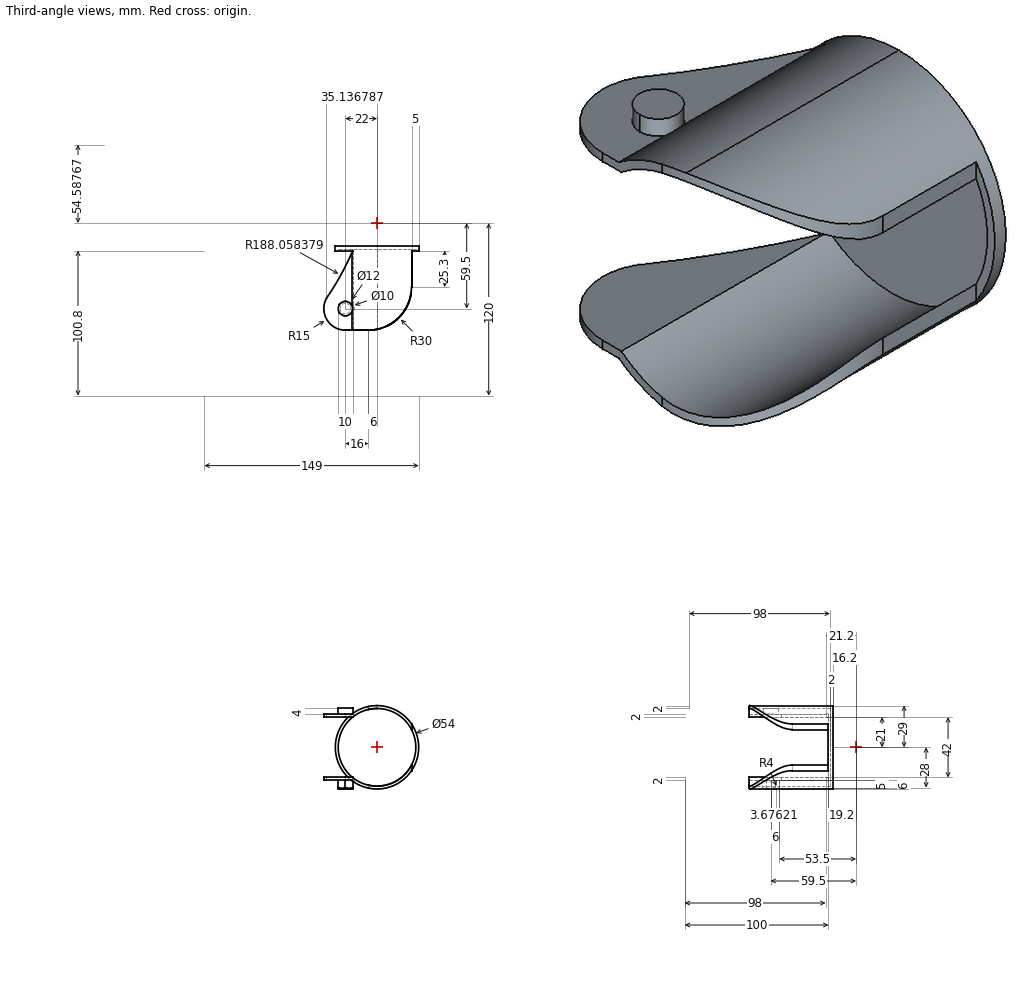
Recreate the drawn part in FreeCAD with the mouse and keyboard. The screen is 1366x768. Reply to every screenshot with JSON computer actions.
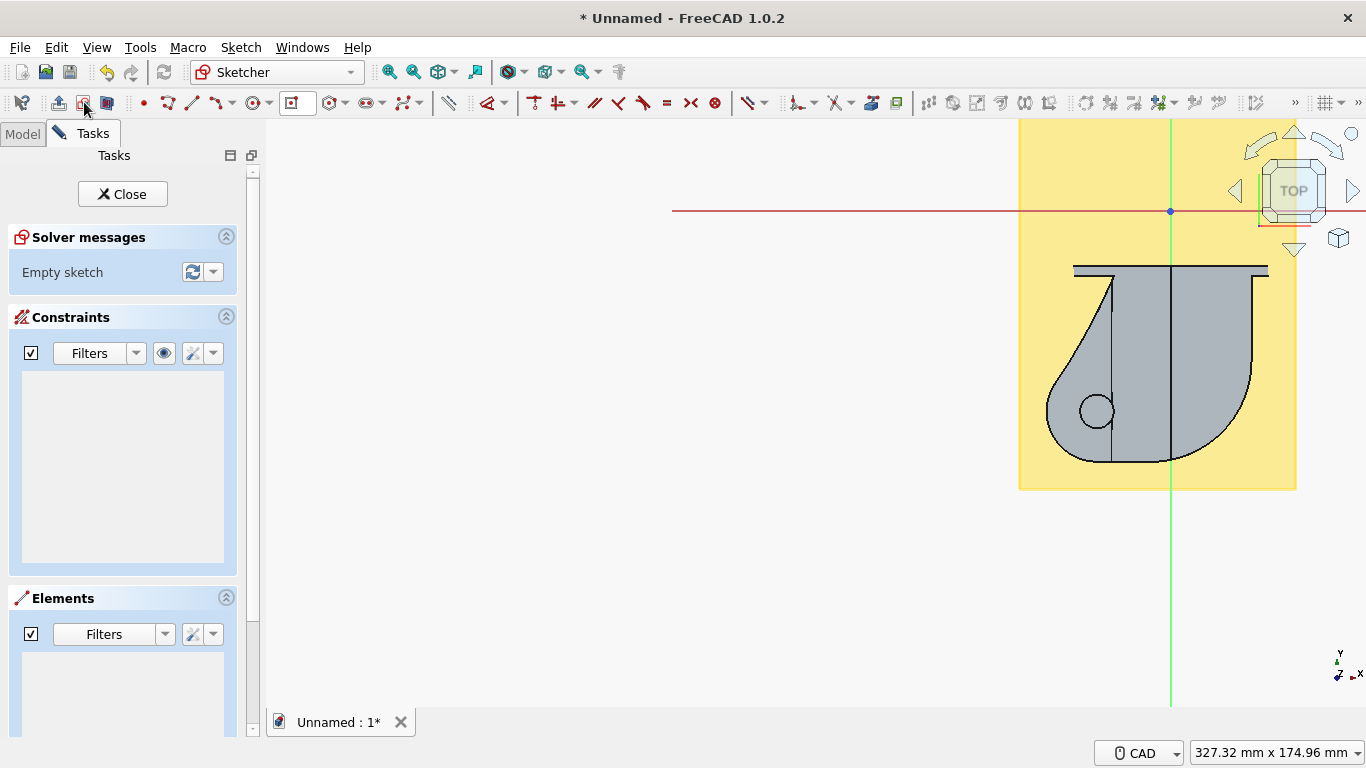
{"action": "left_click", "coordinate": [108, 104]}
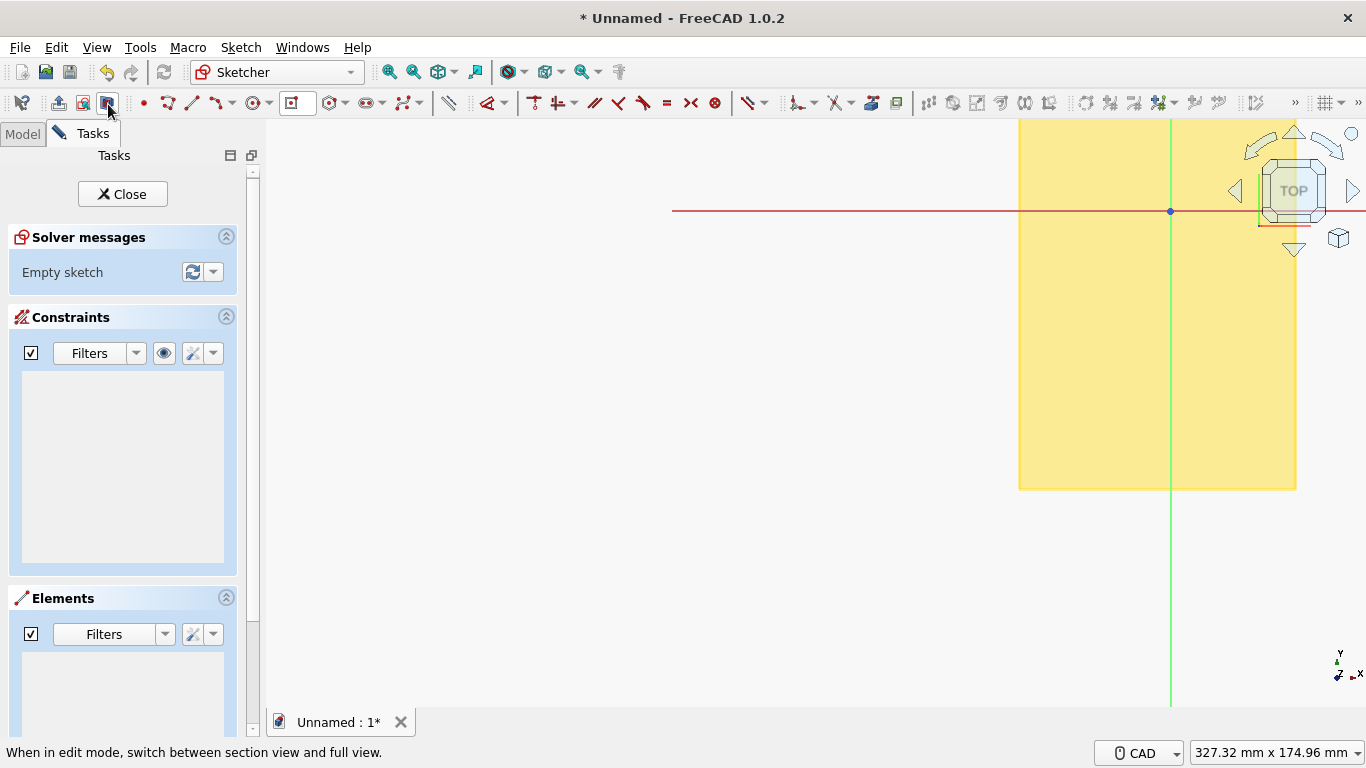
{"action": "scroll", "coordinate": [1140, 411], "scroll_direction": "up", "scroll_amount": 11}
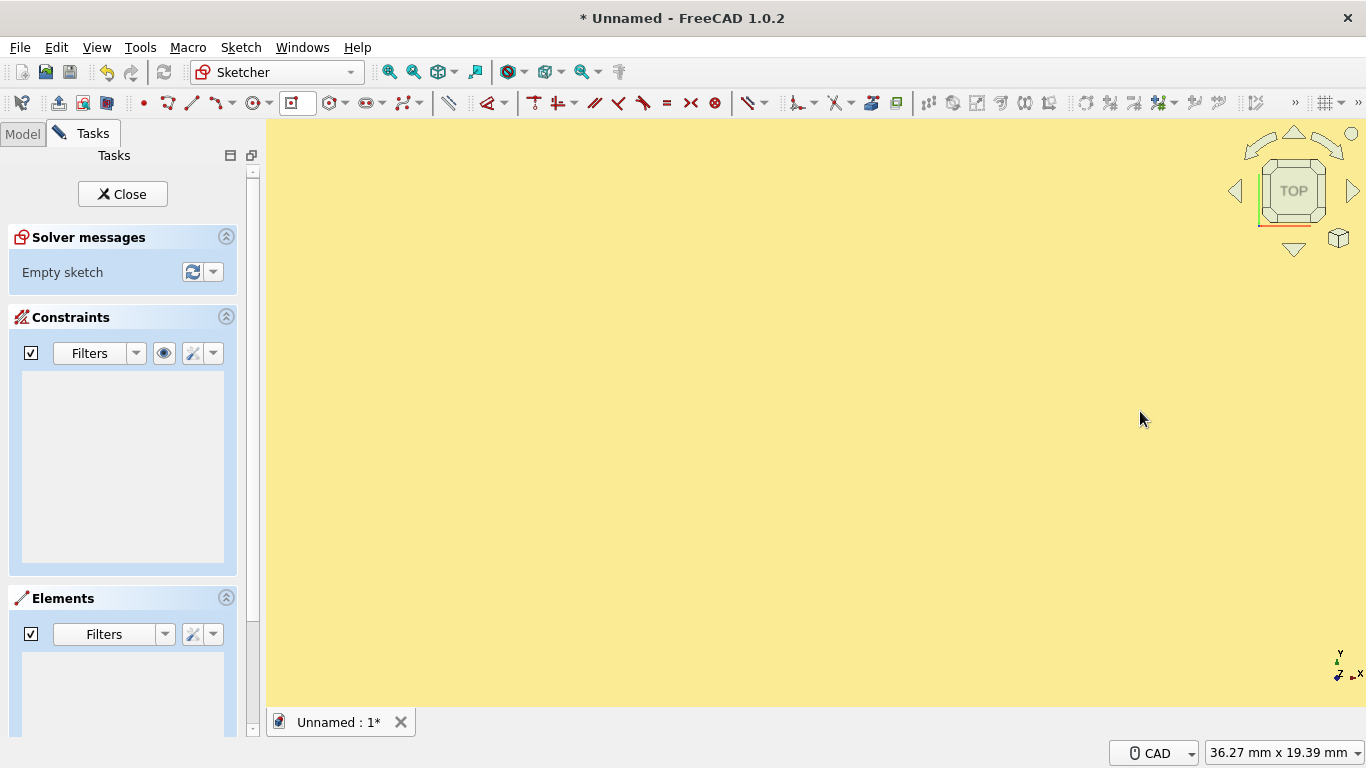
{"action": "left_click", "coordinate": [330, 104]}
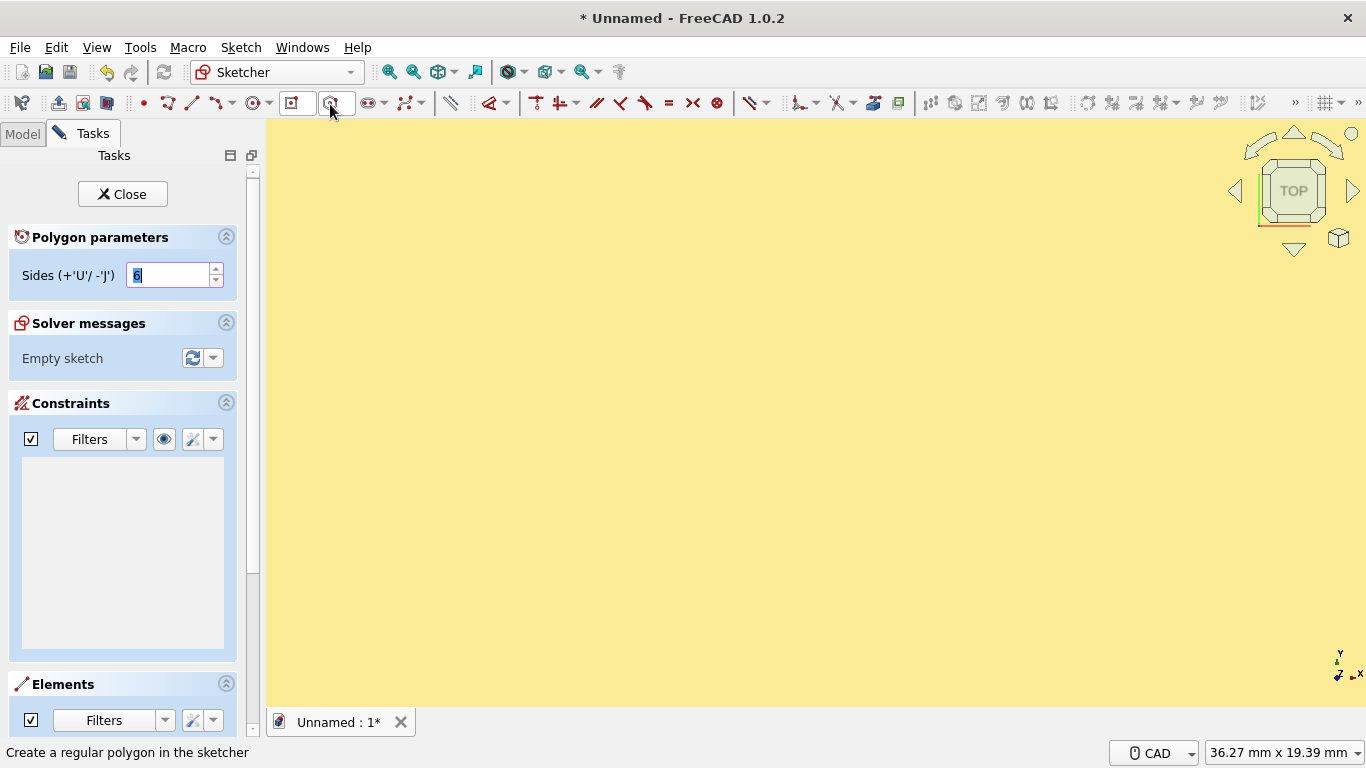
{"action": "left_click", "coordinate": [745, 411]}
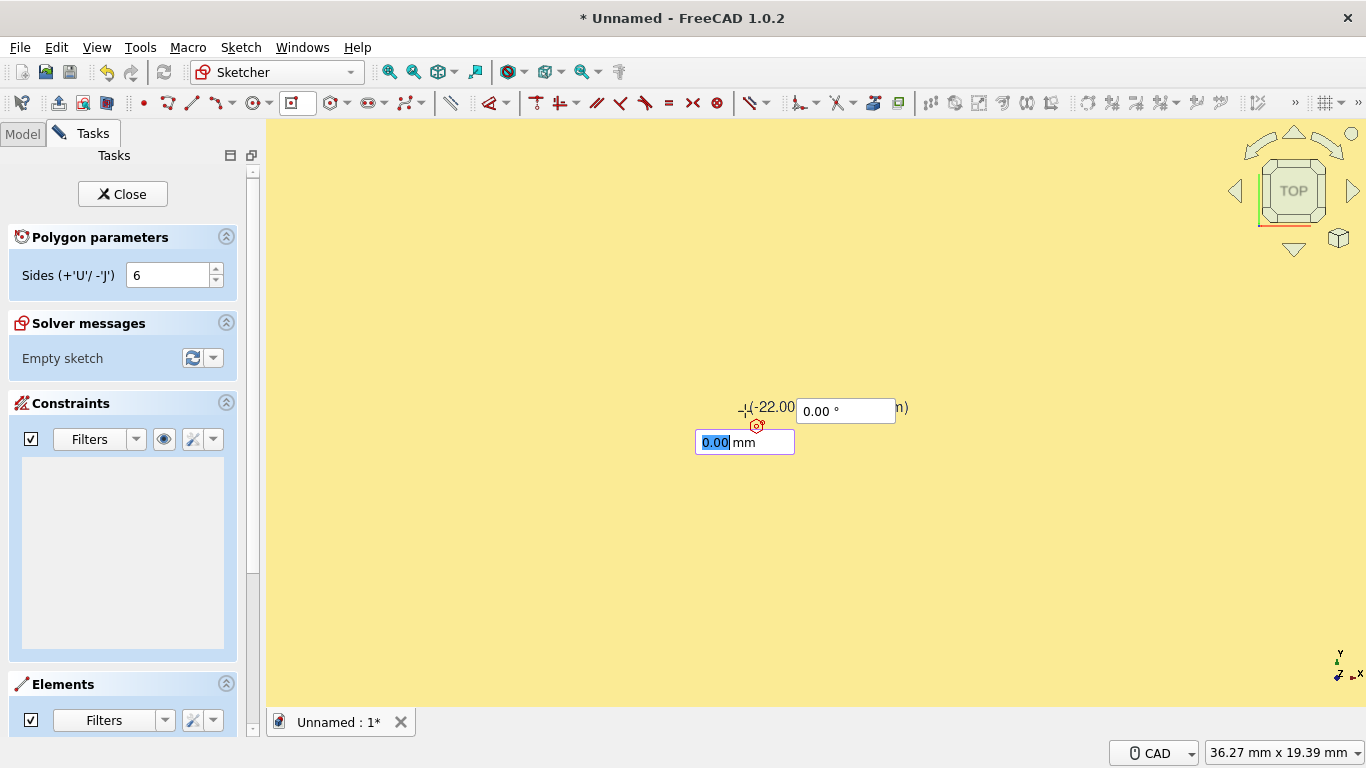
{"action": "left_click", "coordinate": [745, 236]}
{"action": "key", "text": "Escape"}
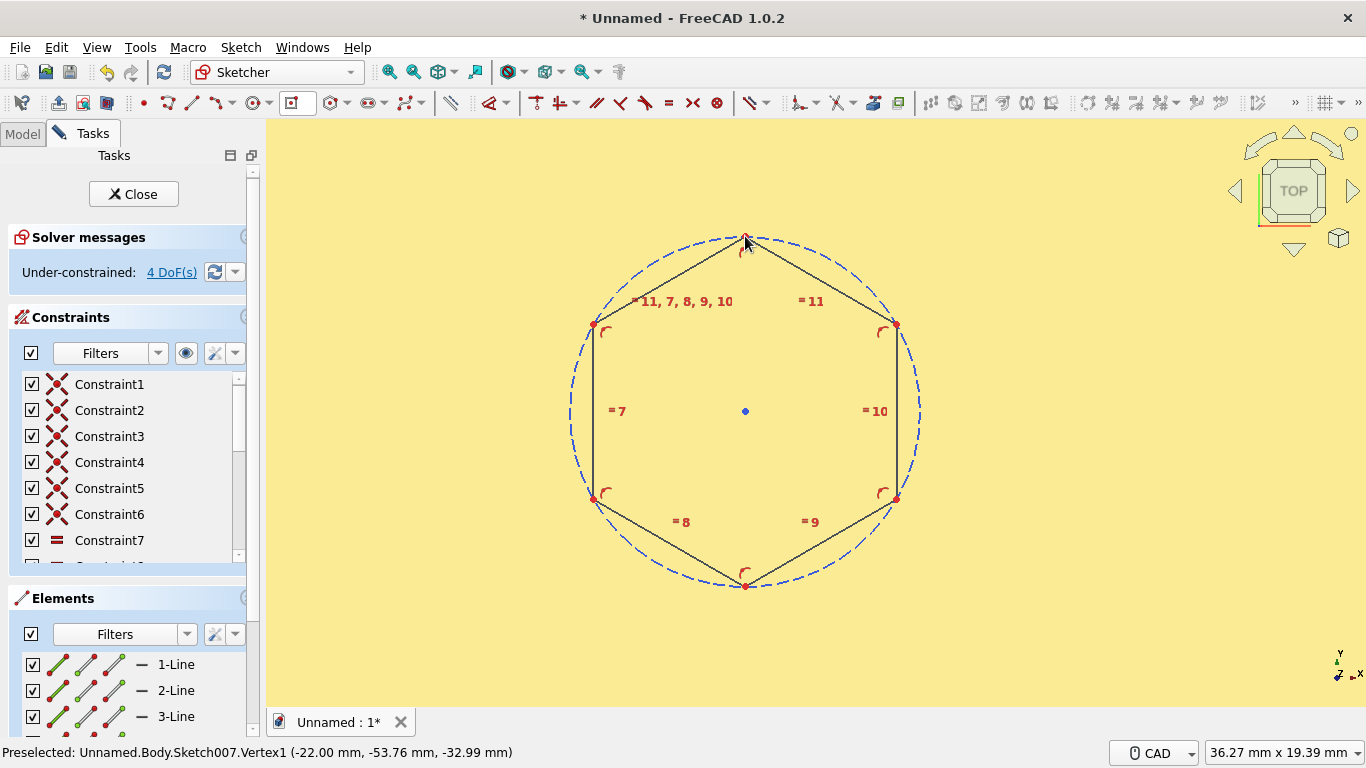
{"action": "left_click", "coordinate": [254, 104]}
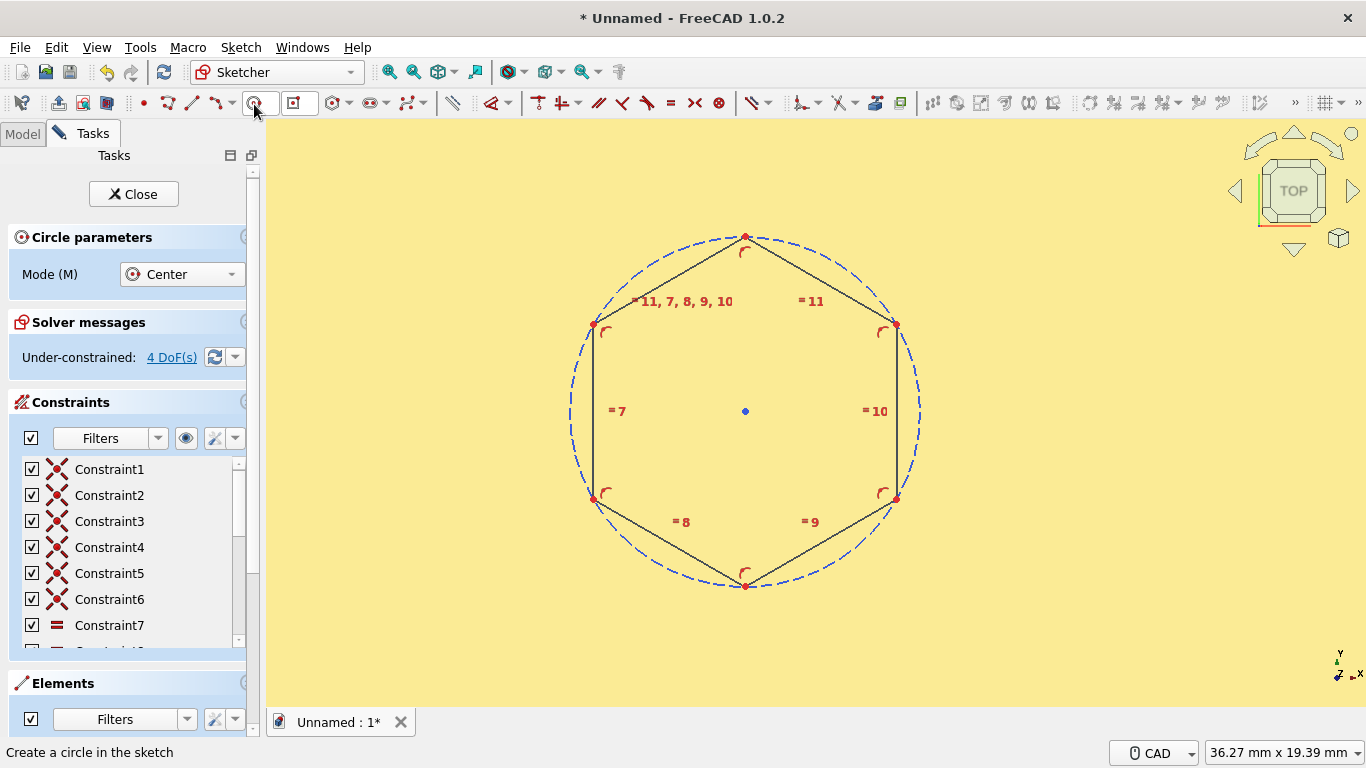
{"action": "left_click", "coordinate": [745, 412]}
{"action": "left_click", "coordinate": [874, 282]}
{"action": "key", "text": "Escape"}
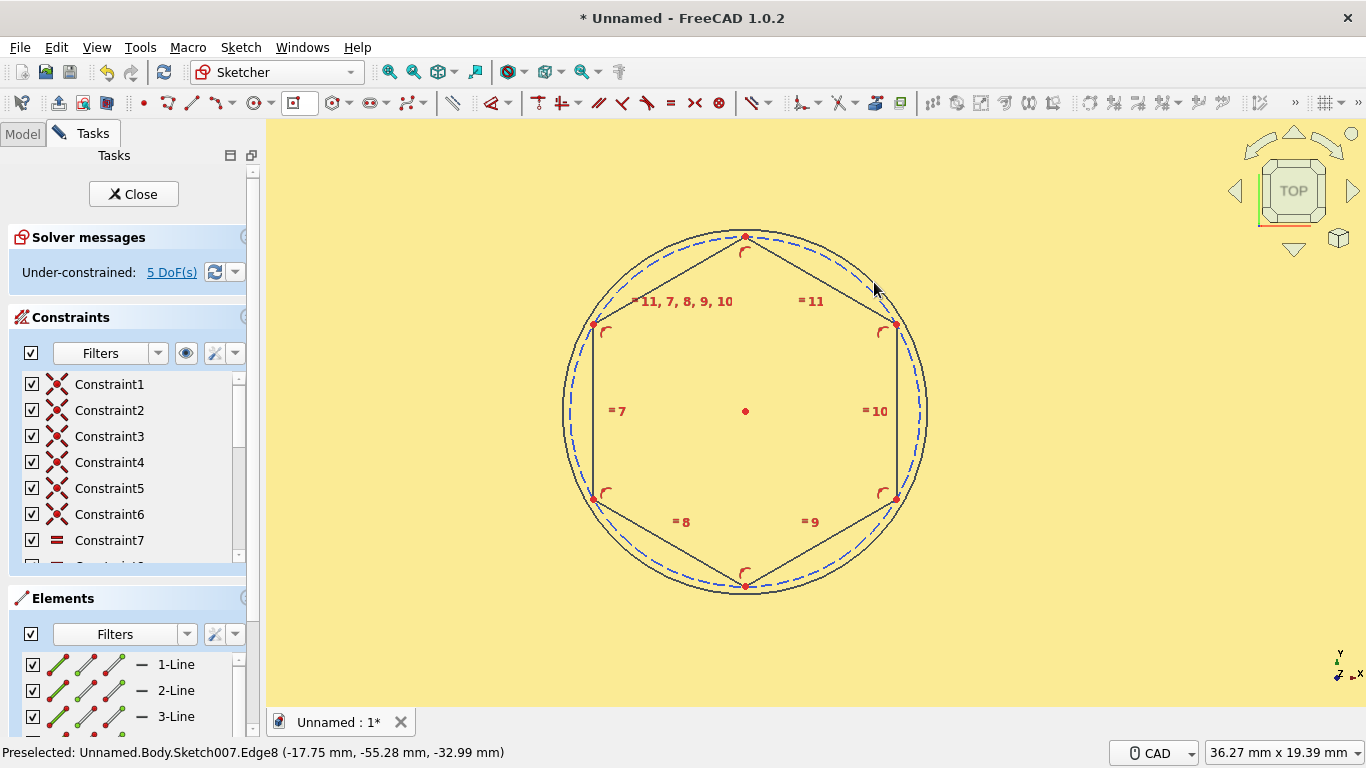
{"action": "left_click", "coordinate": [593, 377]}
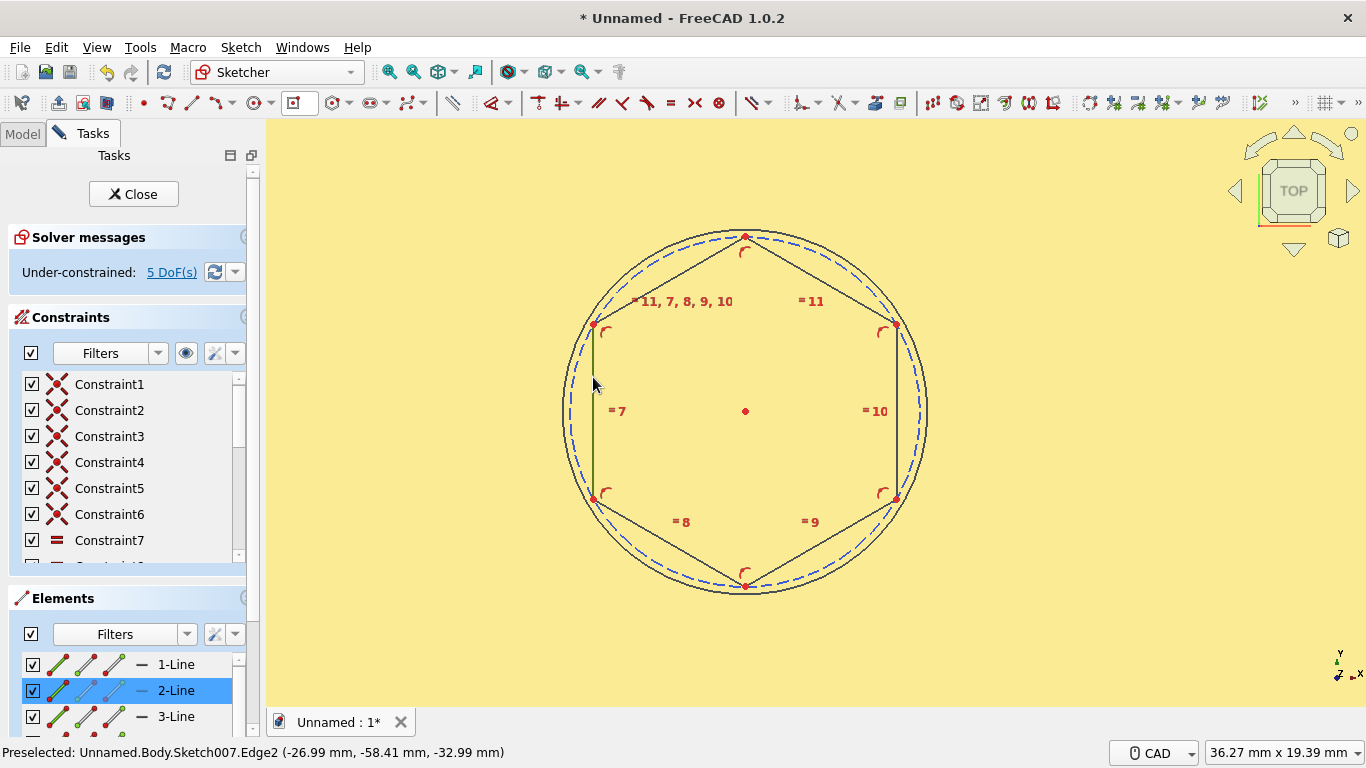
{"action": "left_click", "coordinate": [580, 104]}